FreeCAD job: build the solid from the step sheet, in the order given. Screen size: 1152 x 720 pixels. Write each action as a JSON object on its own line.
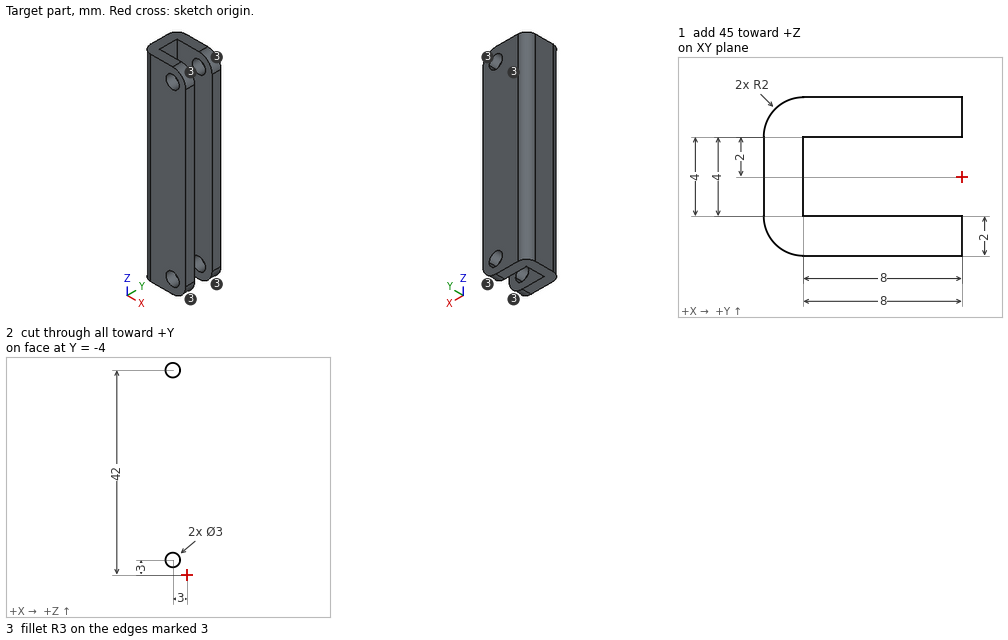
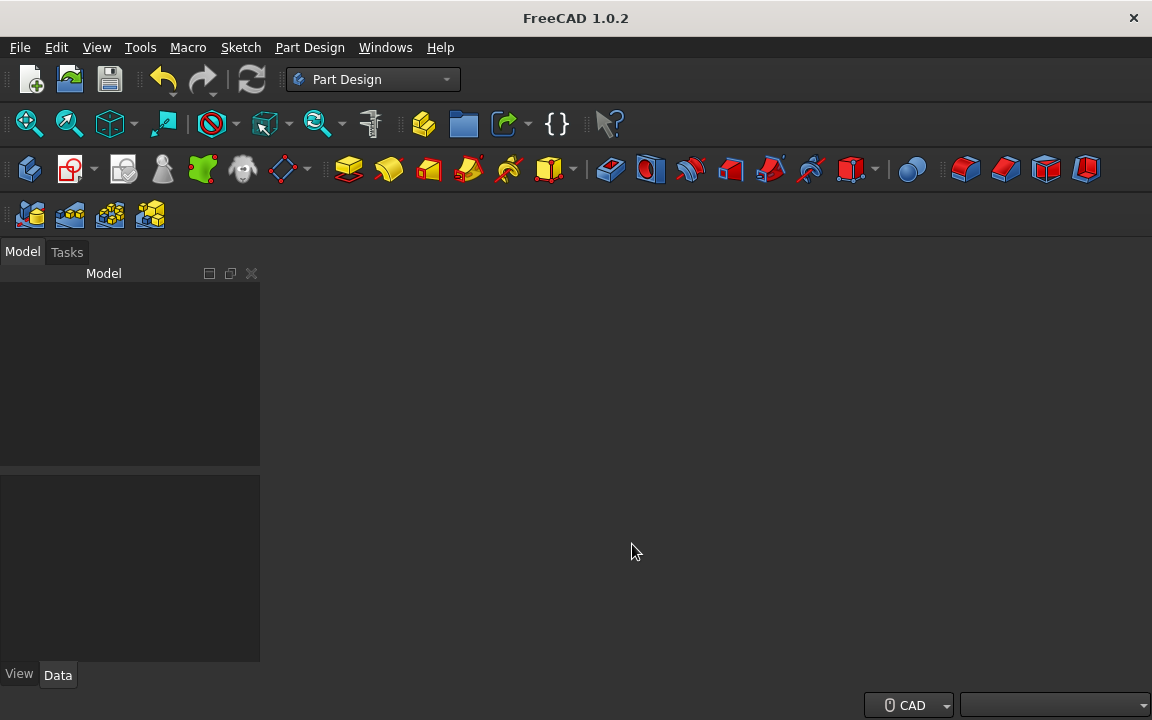
{"action": "left_click", "coordinate": [30, 80]}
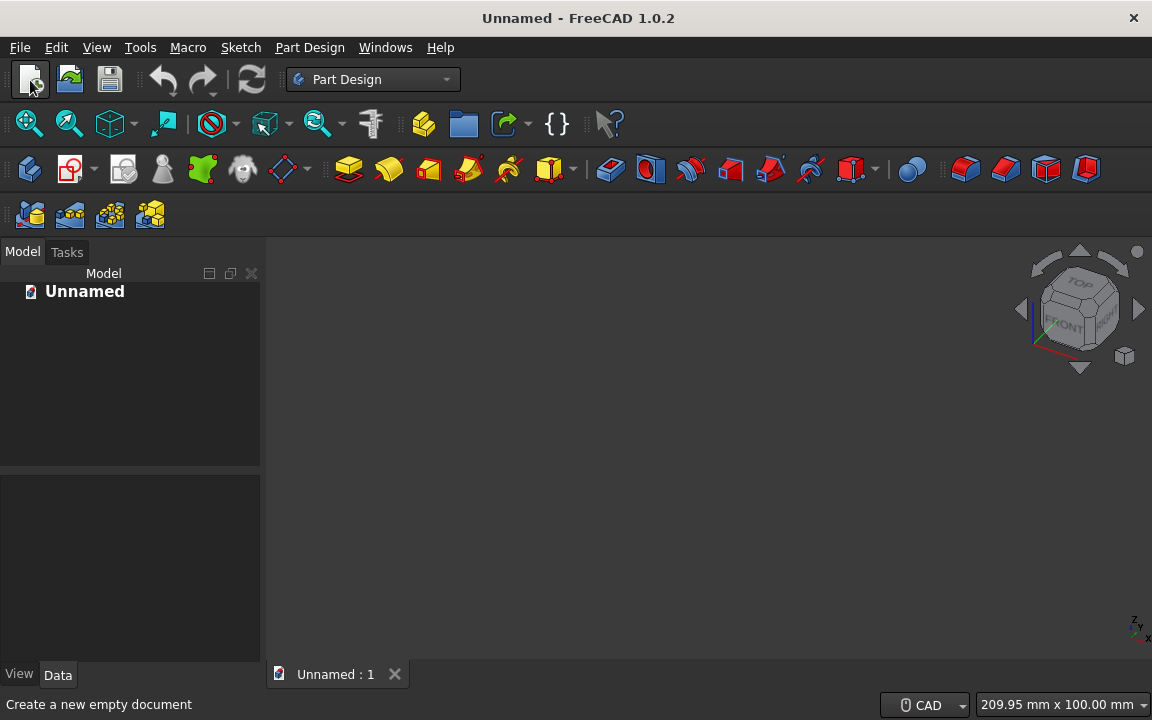
{"action": "left_click", "coordinate": [70, 170]}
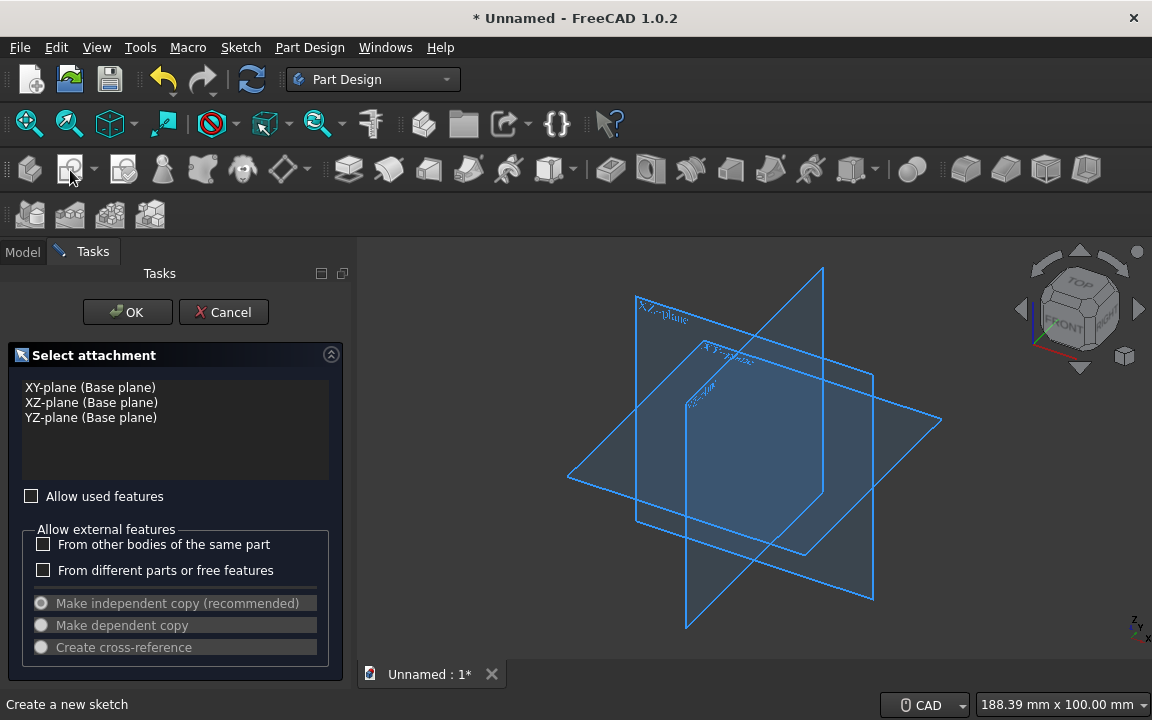
{"action": "left_click", "coordinate": [82, 388]}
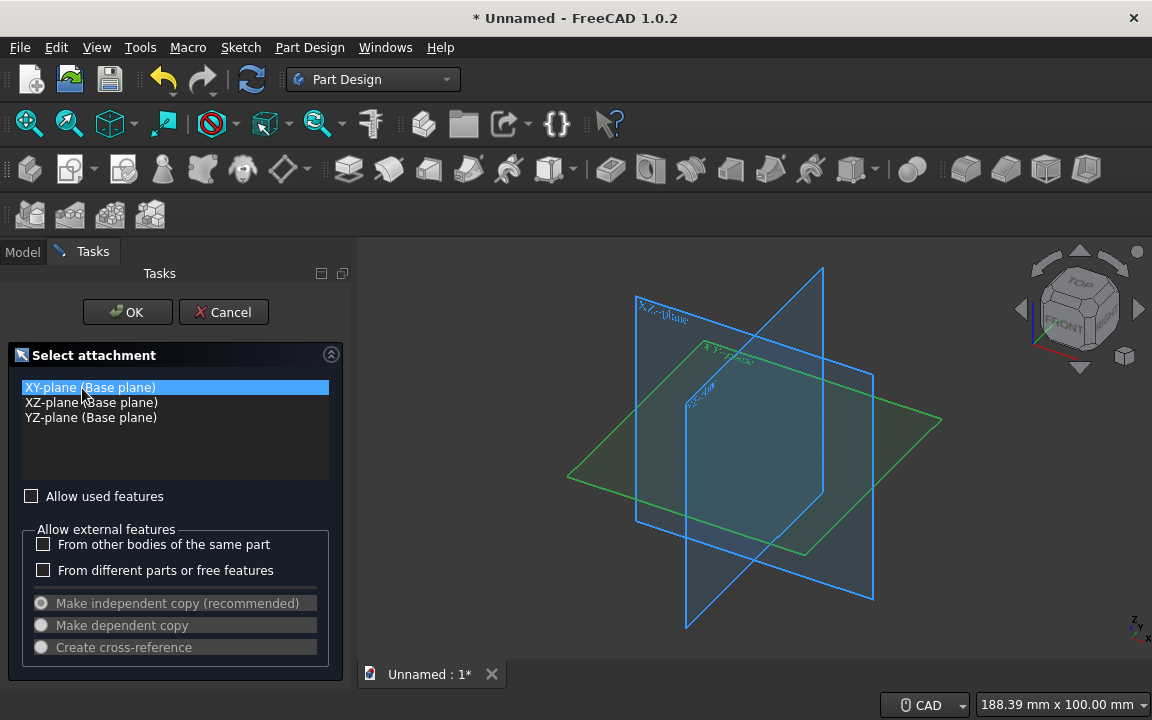
{"action": "left_click", "coordinate": [128, 312]}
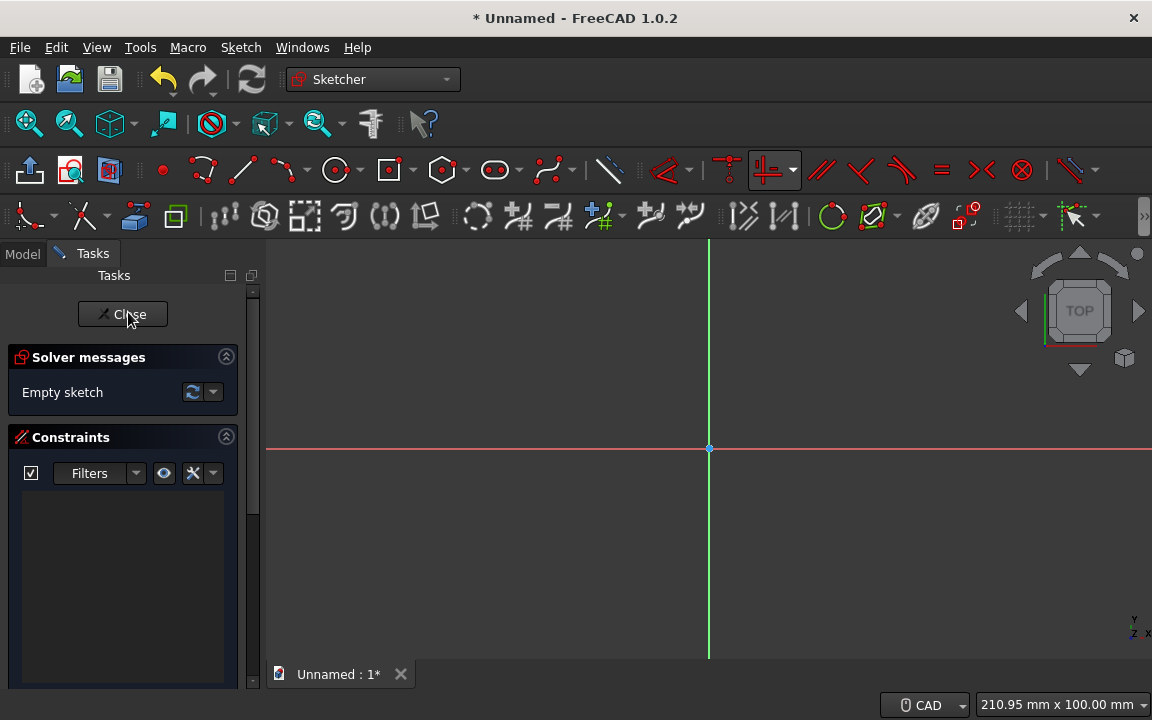
{"action": "scroll", "coordinate": [695, 449], "scroll_direction": "up", "scroll_amount": 10}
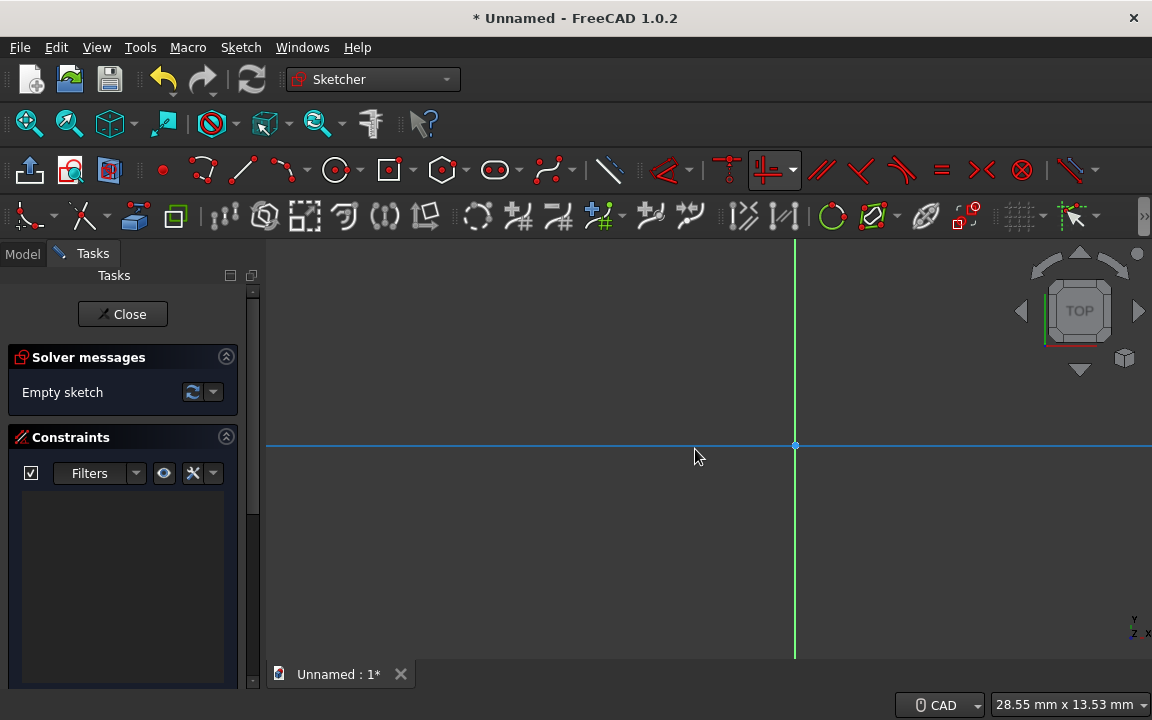
{"action": "left_click", "coordinate": [244, 170]}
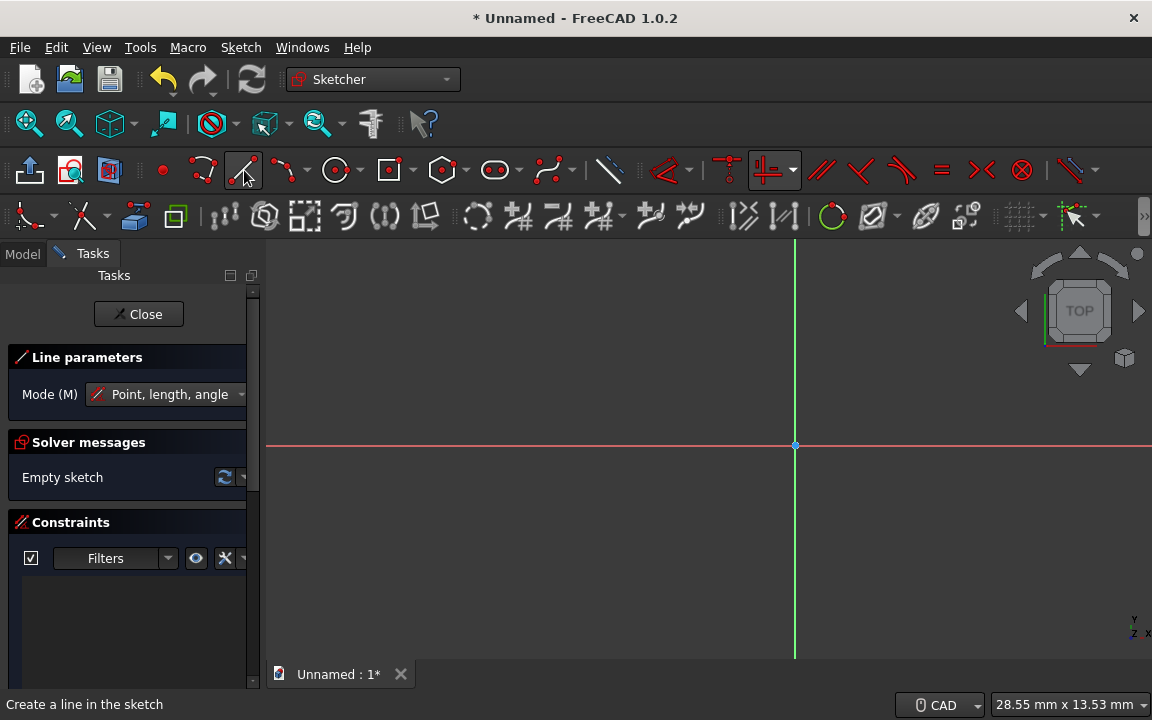
{"action": "left_click", "coordinate": [485, 384]}
{"action": "left_click", "coordinate": [485, 508]}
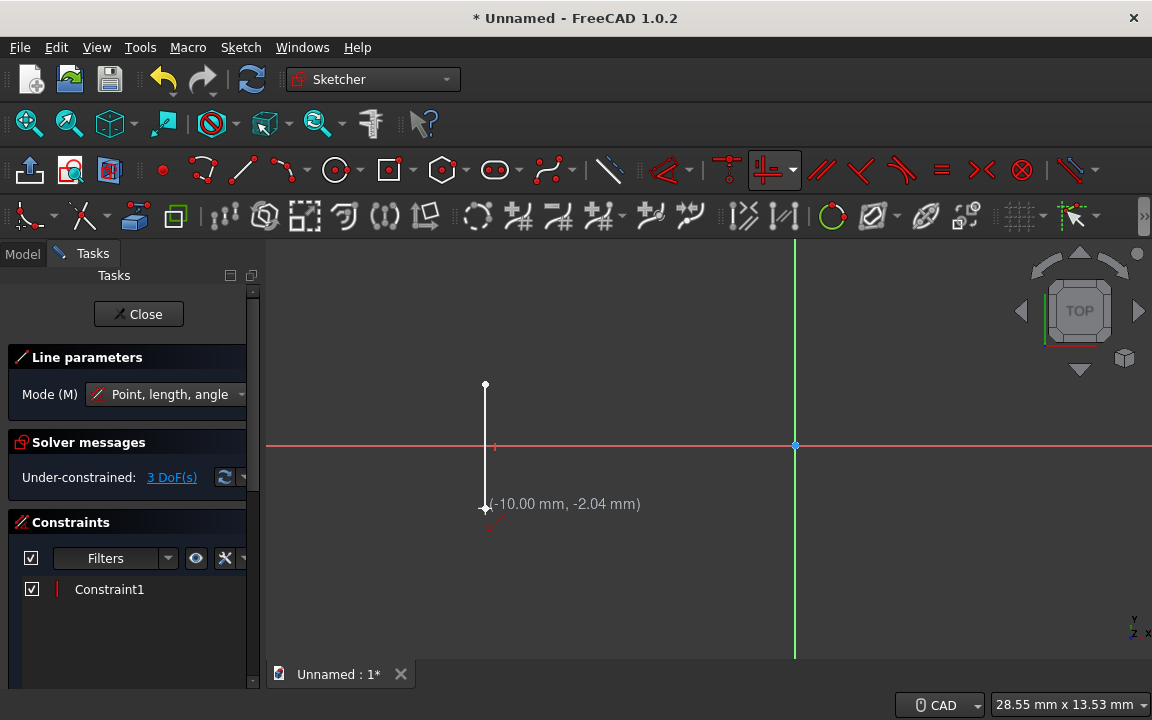
{"action": "left_click", "coordinate": [204, 170]}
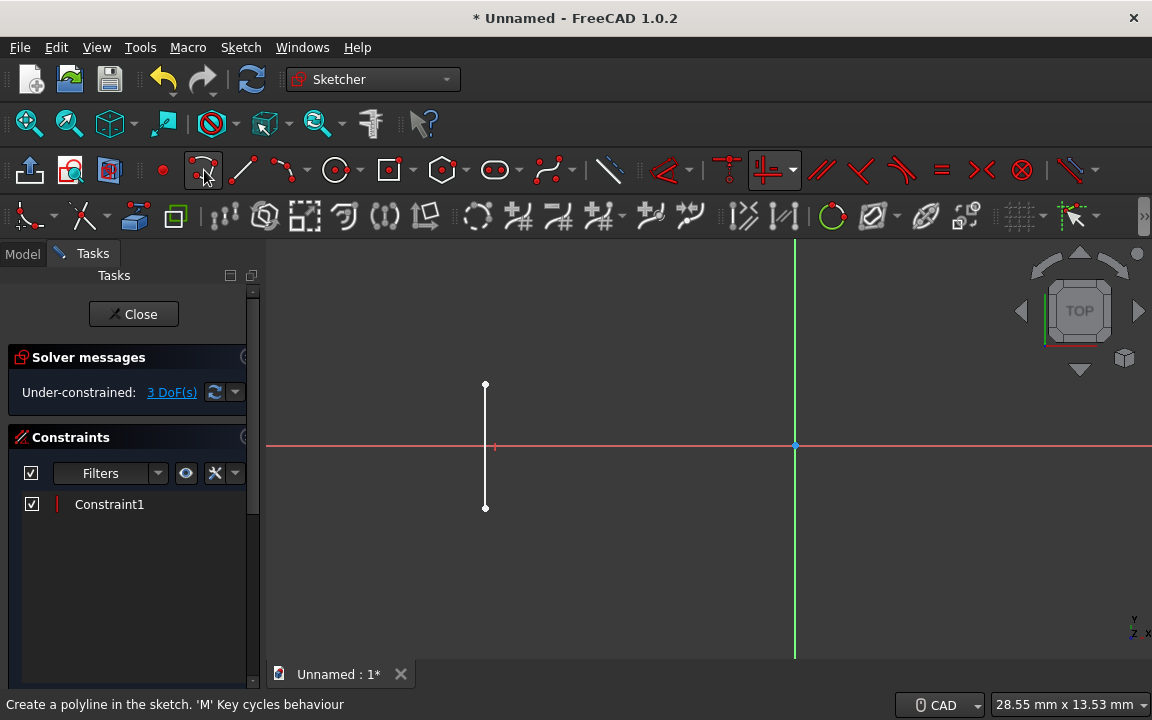
{"action": "left_click", "coordinate": [547, 570]}
{"action": "left_click", "coordinate": [795, 570]}
{"action": "left_click", "coordinate": [786, 508]}
{"action": "left_click", "coordinate": [547, 508]}
{"action": "left_click", "coordinate": [547, 384]}
{"action": "left_click", "coordinate": [795, 384]}
{"action": "left_click", "coordinate": [786, 322]}
{"action": "left_click", "coordinate": [547, 322]}
{"action": "right_click", "coordinate": [547, 322]}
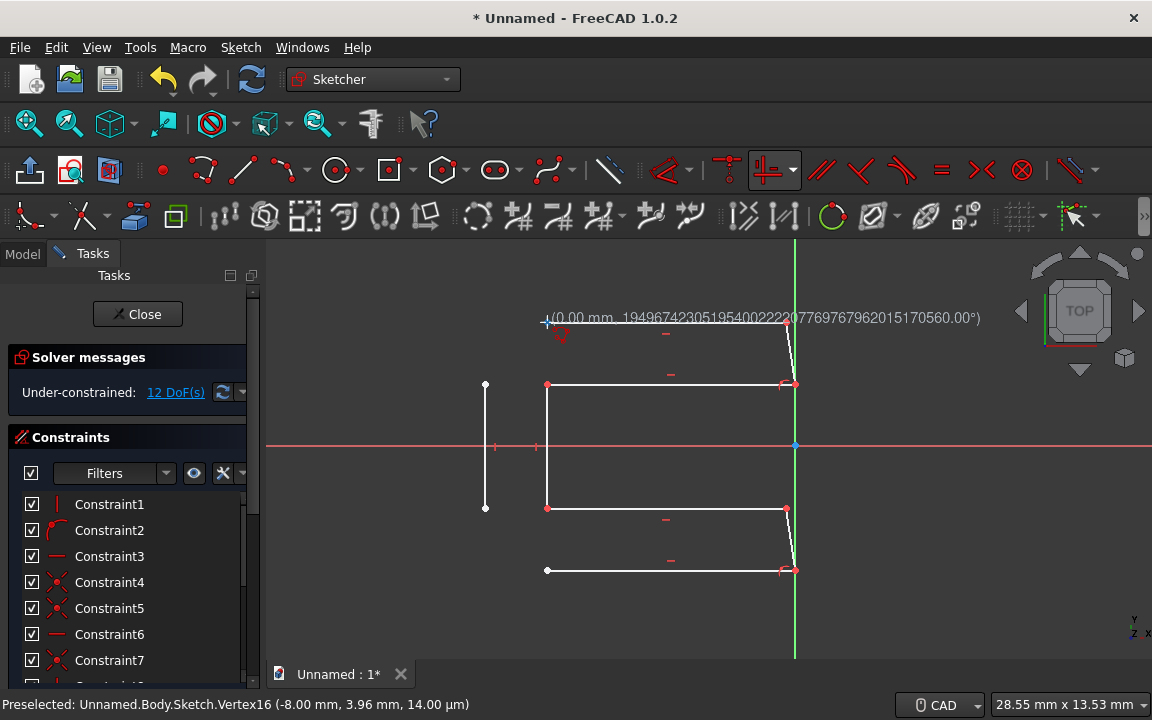
{"action": "left_click", "coordinate": [284, 170]}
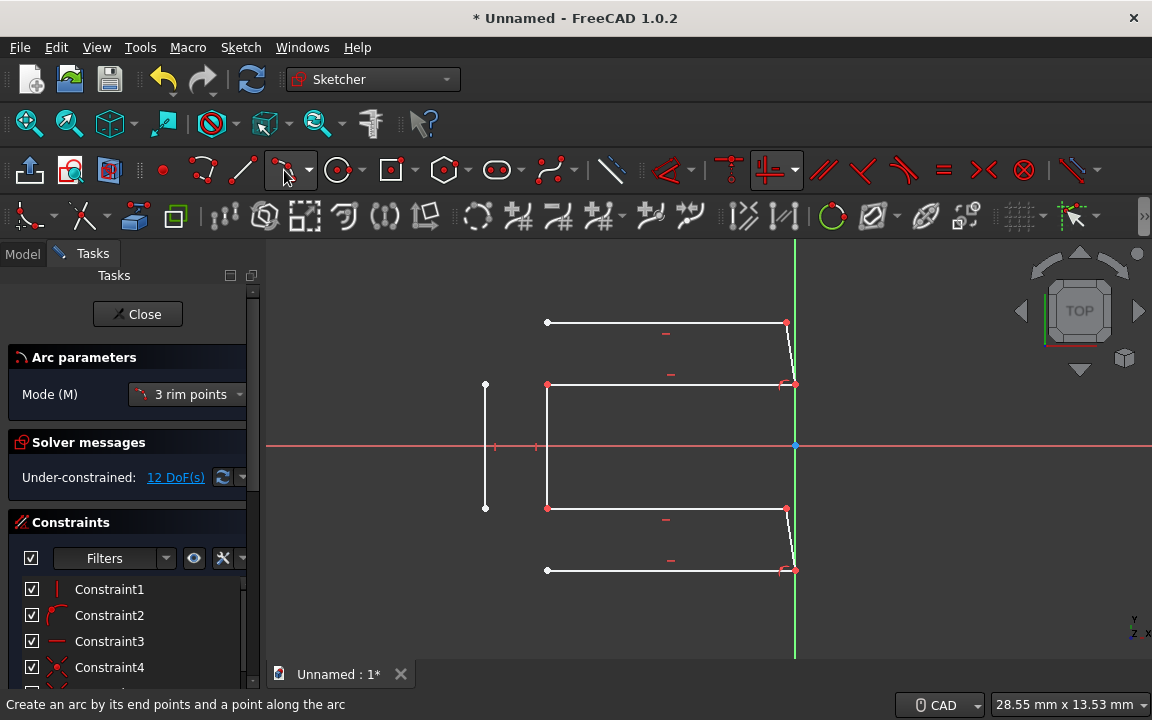
{"action": "left_click", "coordinate": [485, 509]}
{"action": "left_click", "coordinate": [547, 571]}
{"action": "left_click", "coordinate": [503, 552]}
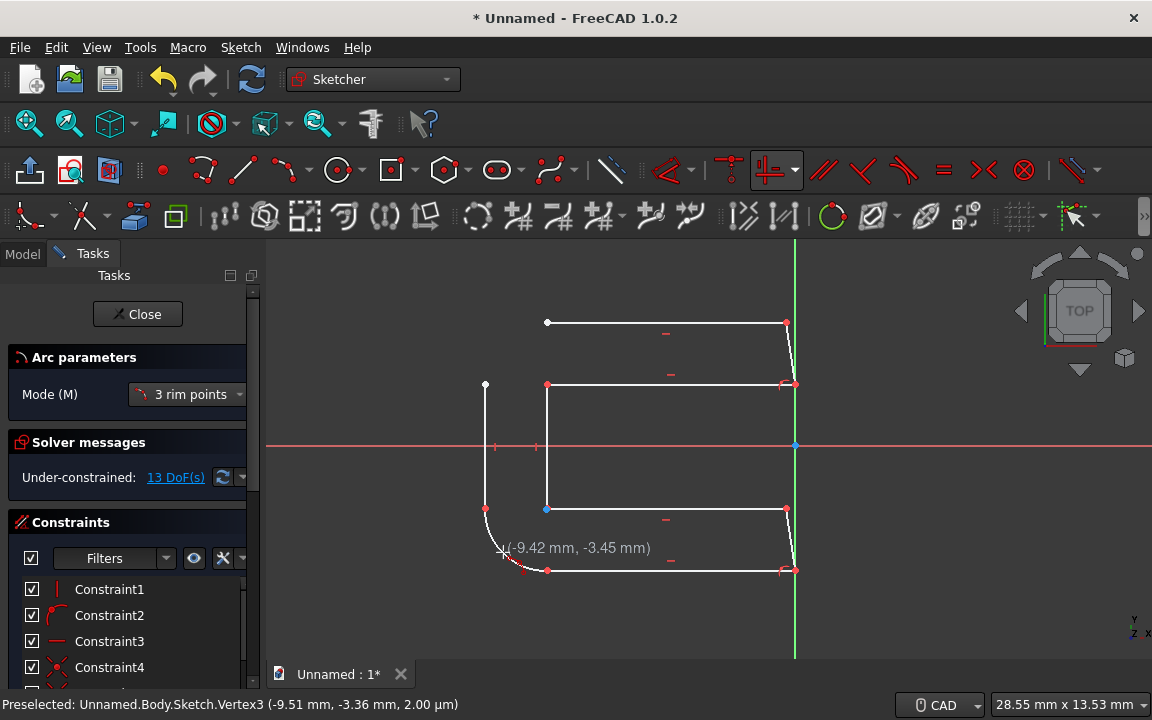
{"action": "left_click", "coordinate": [547, 323]}
{"action": "left_click", "coordinate": [485, 385]}
{"action": "left_click", "coordinate": [503, 340]}
{"action": "key", "text": "Escape"}